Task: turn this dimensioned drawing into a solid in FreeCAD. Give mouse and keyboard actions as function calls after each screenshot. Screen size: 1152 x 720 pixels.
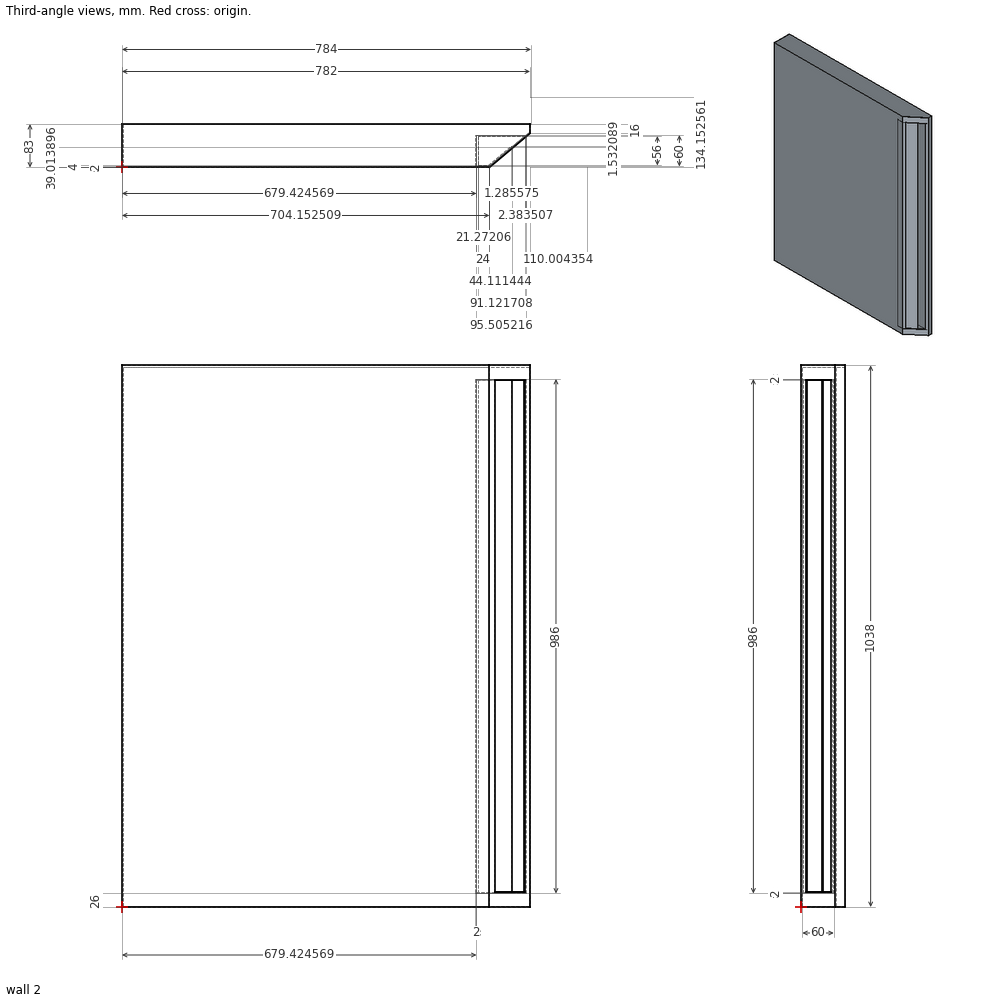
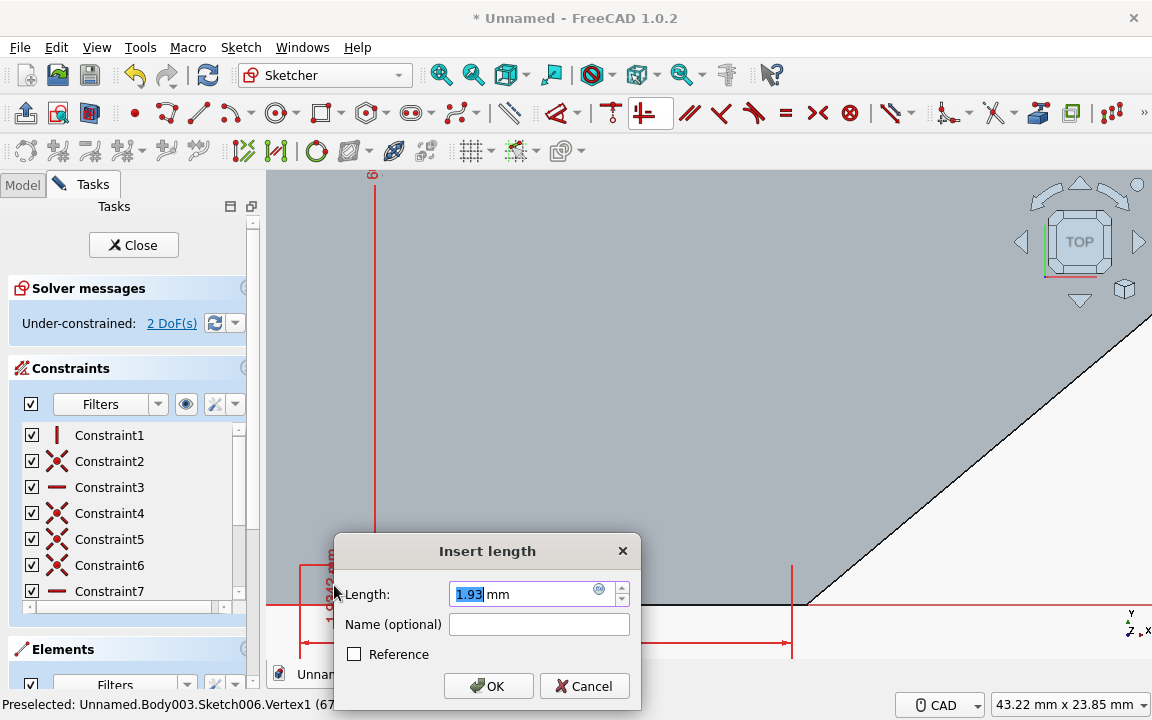
text(2)
key(Return)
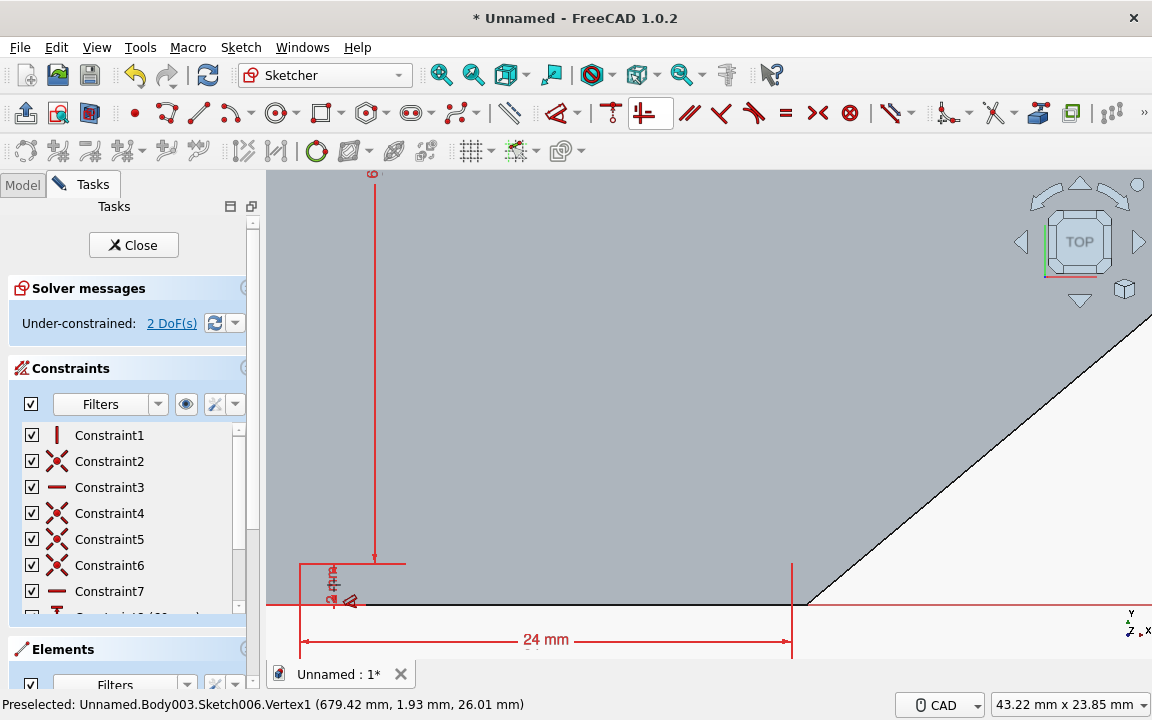
scroll(432, 567, down, 7)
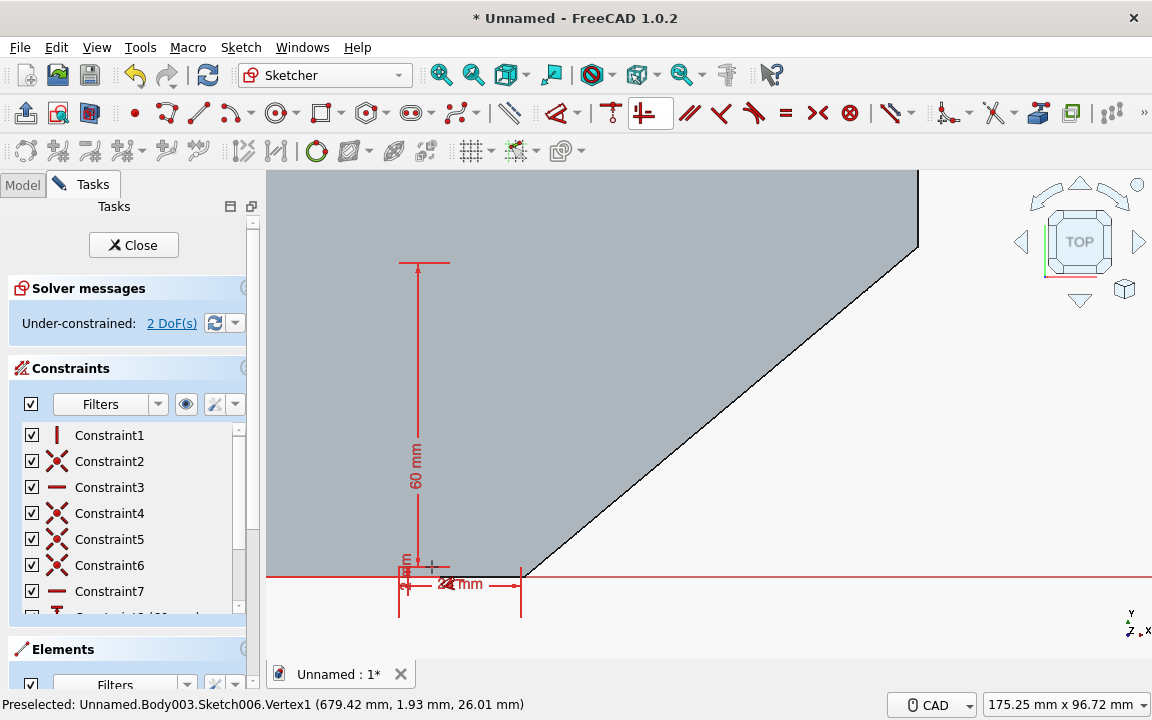
click(544, 263)
click(641, 229)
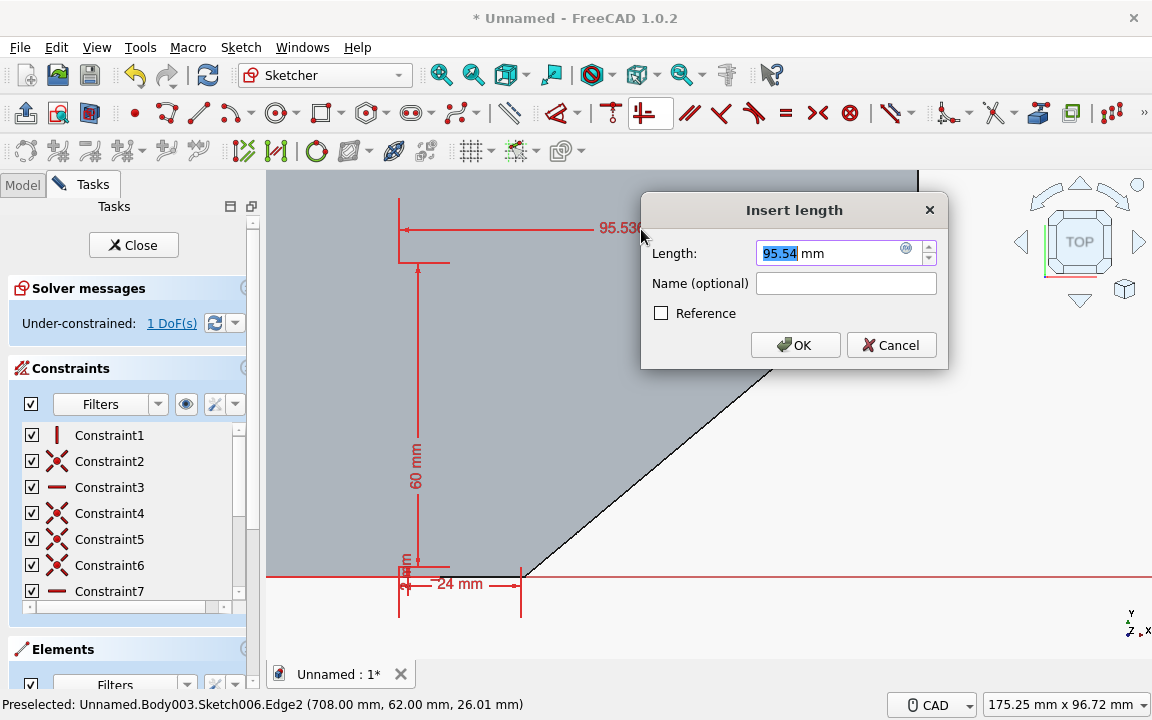
text(95.505216)
key(Return)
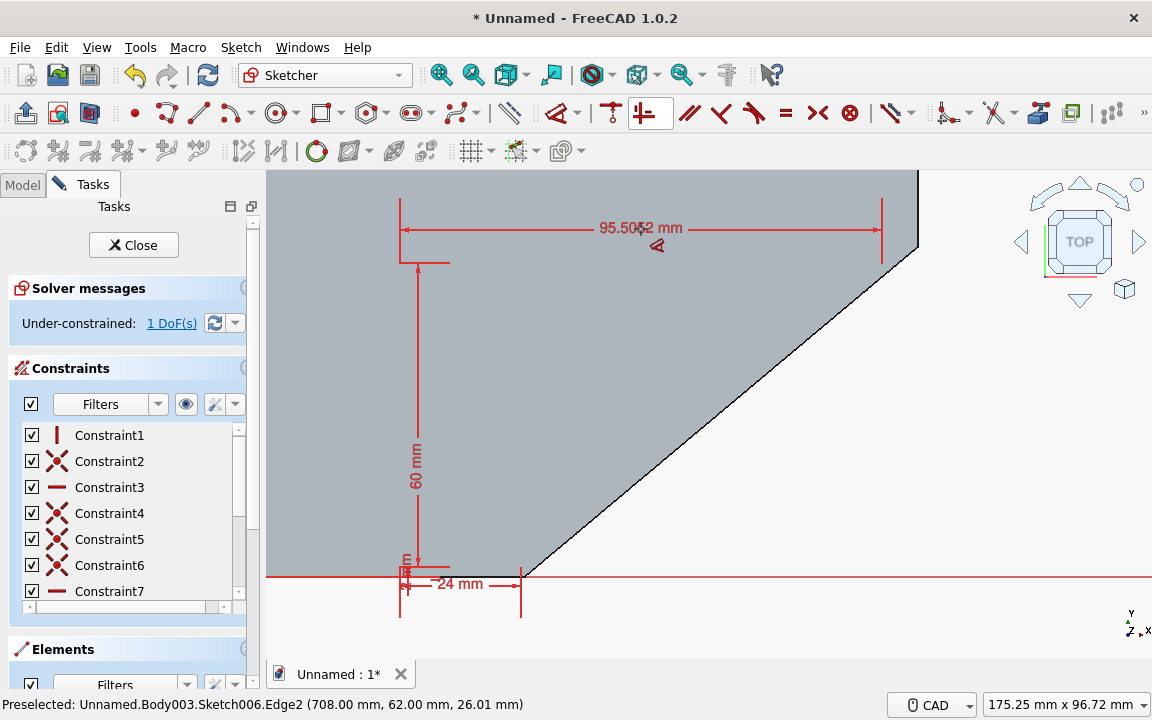
click(400, 567)
click(347, 611)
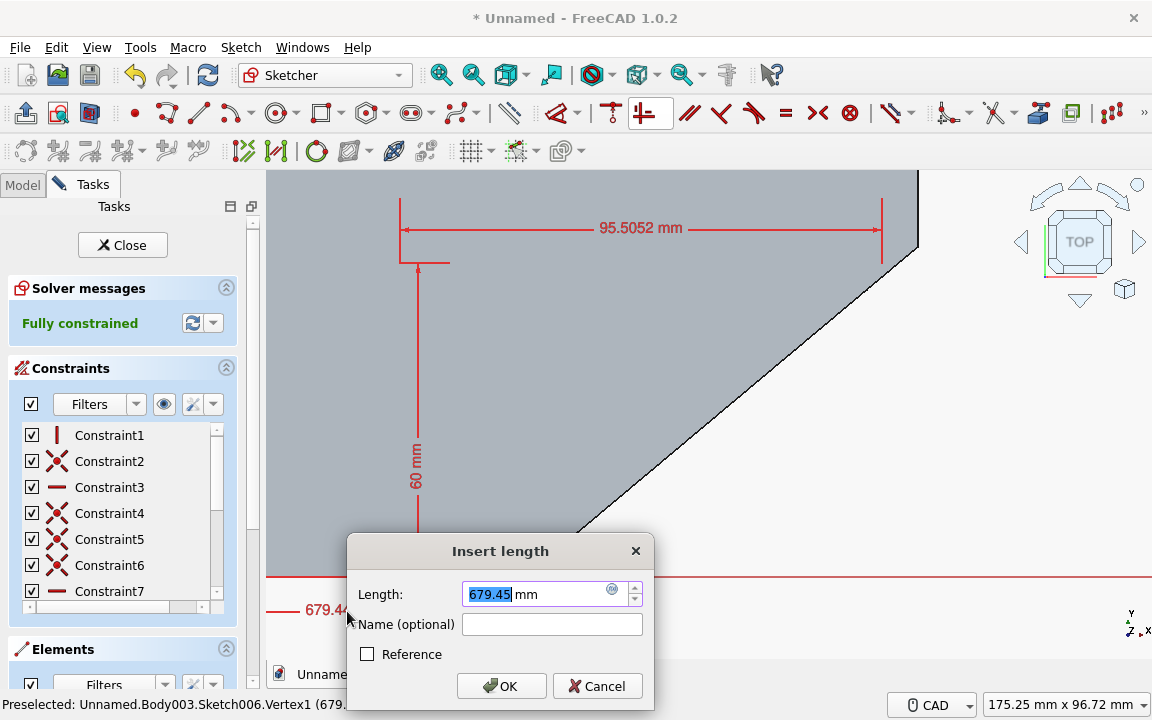
text(679.424569)
key(Return)
key(Escape)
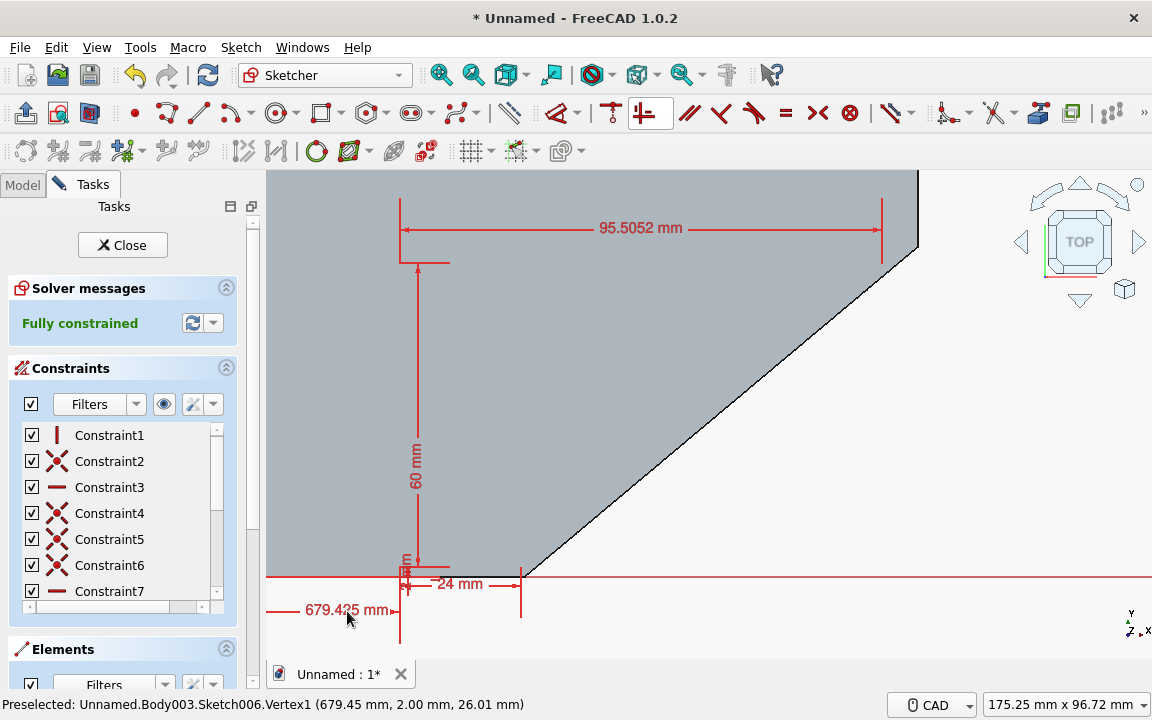
click(123, 245)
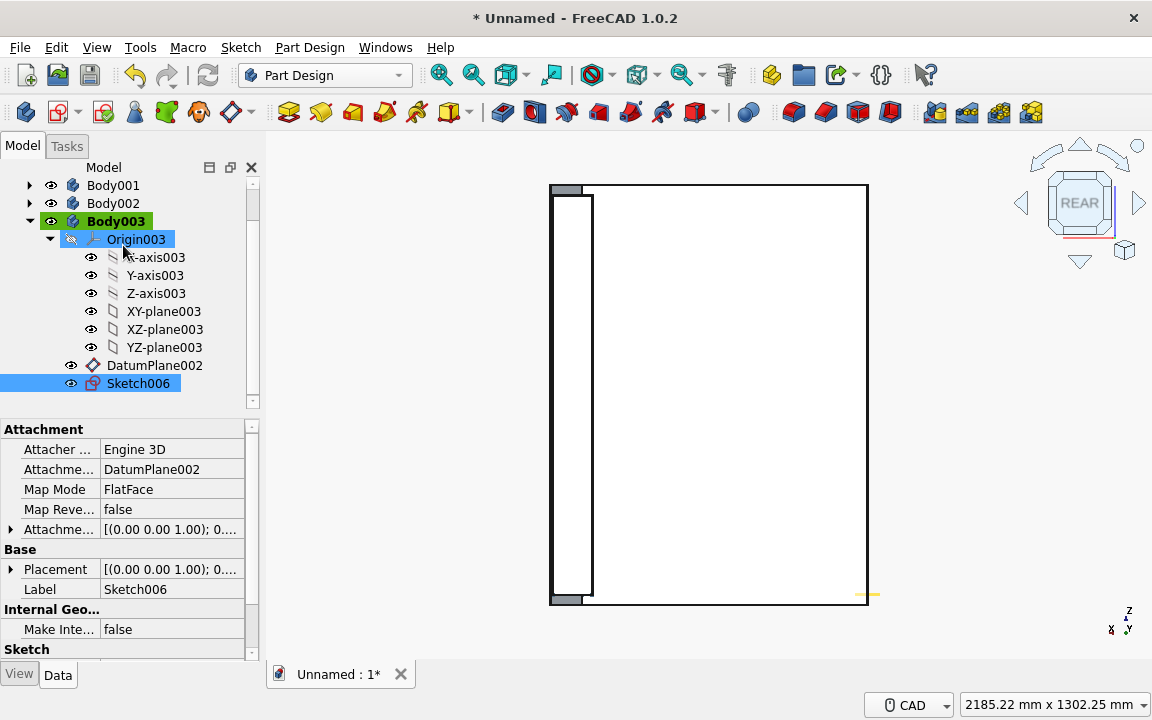
click(290, 112)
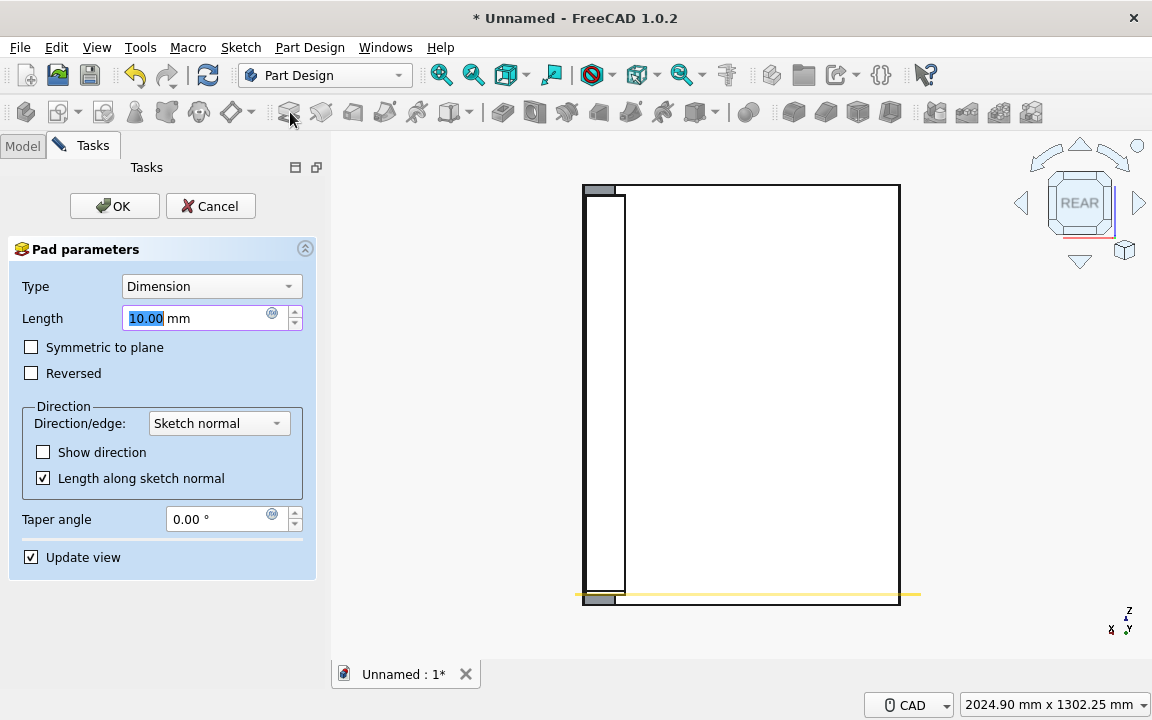
text(2)
key(Tab)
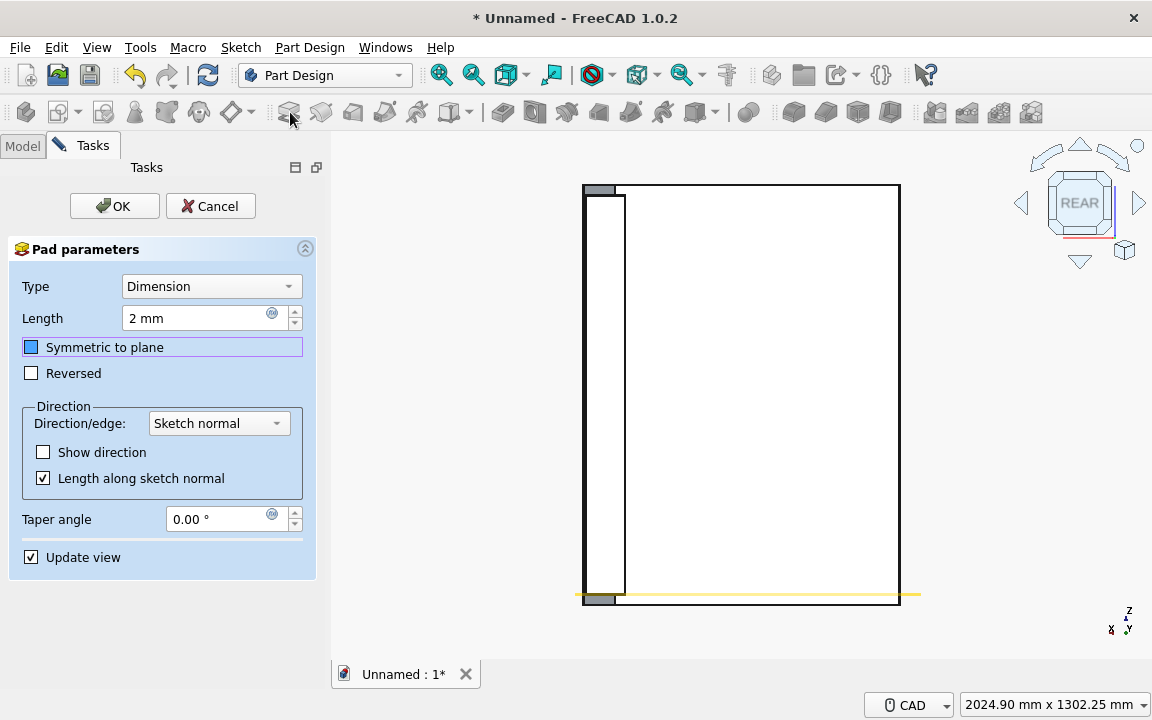
click(115, 206)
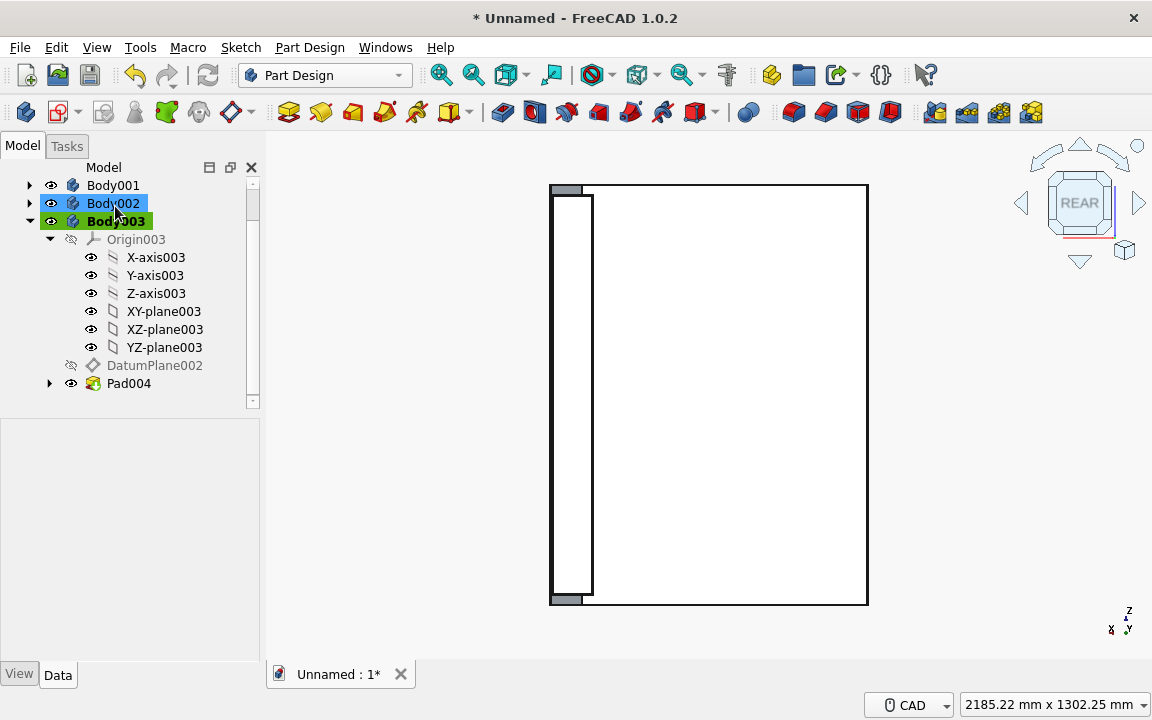
key(0)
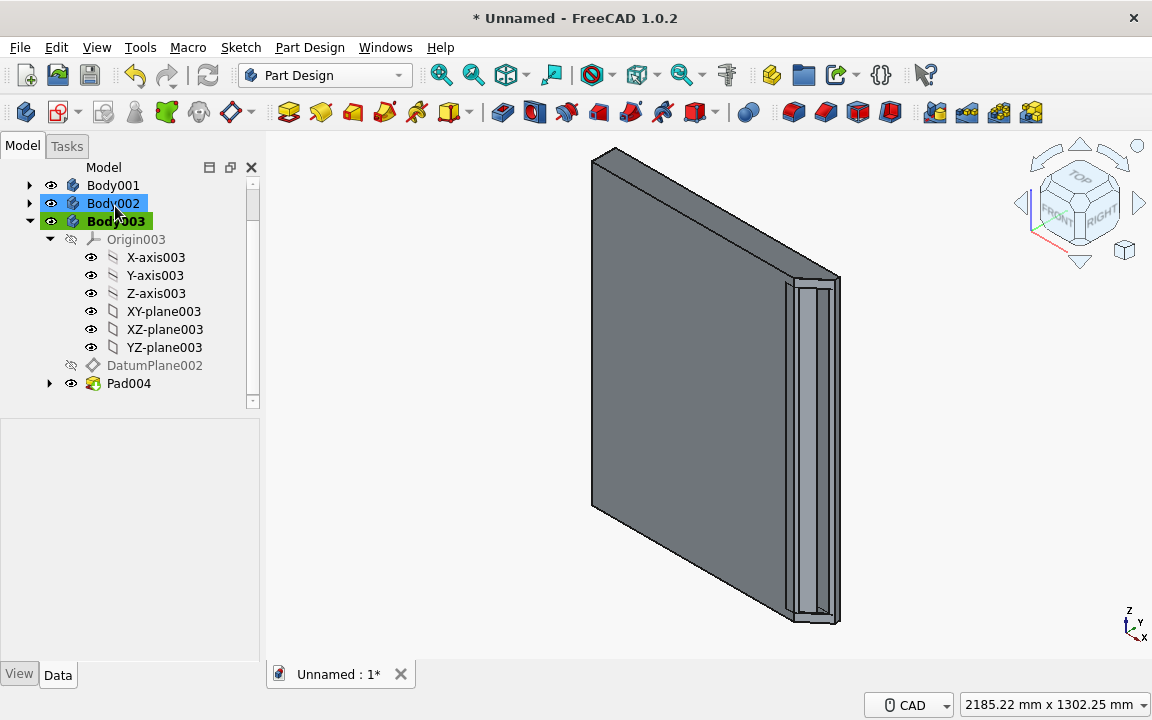
click(442, 76)